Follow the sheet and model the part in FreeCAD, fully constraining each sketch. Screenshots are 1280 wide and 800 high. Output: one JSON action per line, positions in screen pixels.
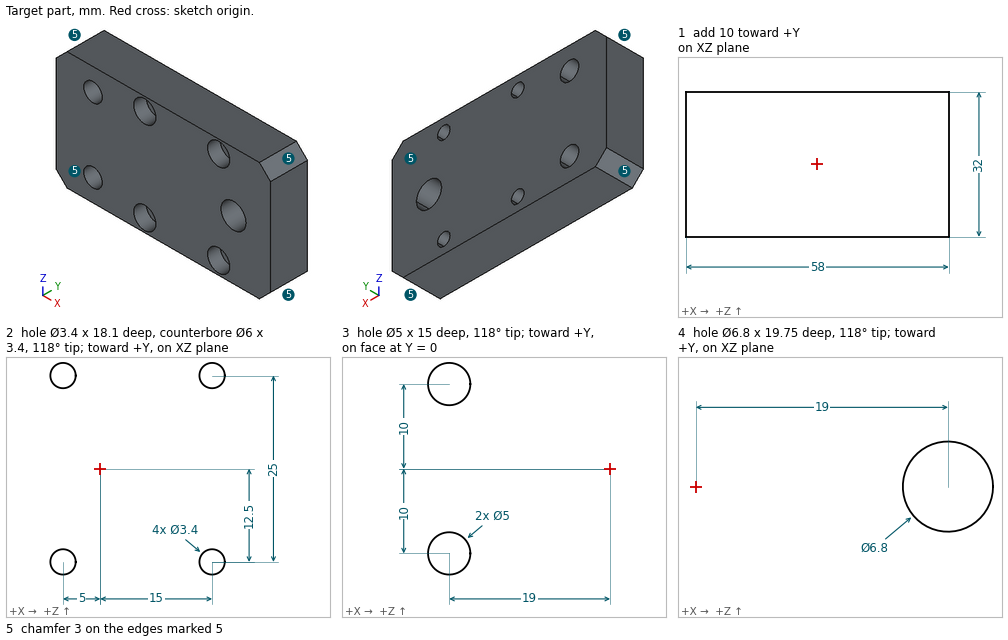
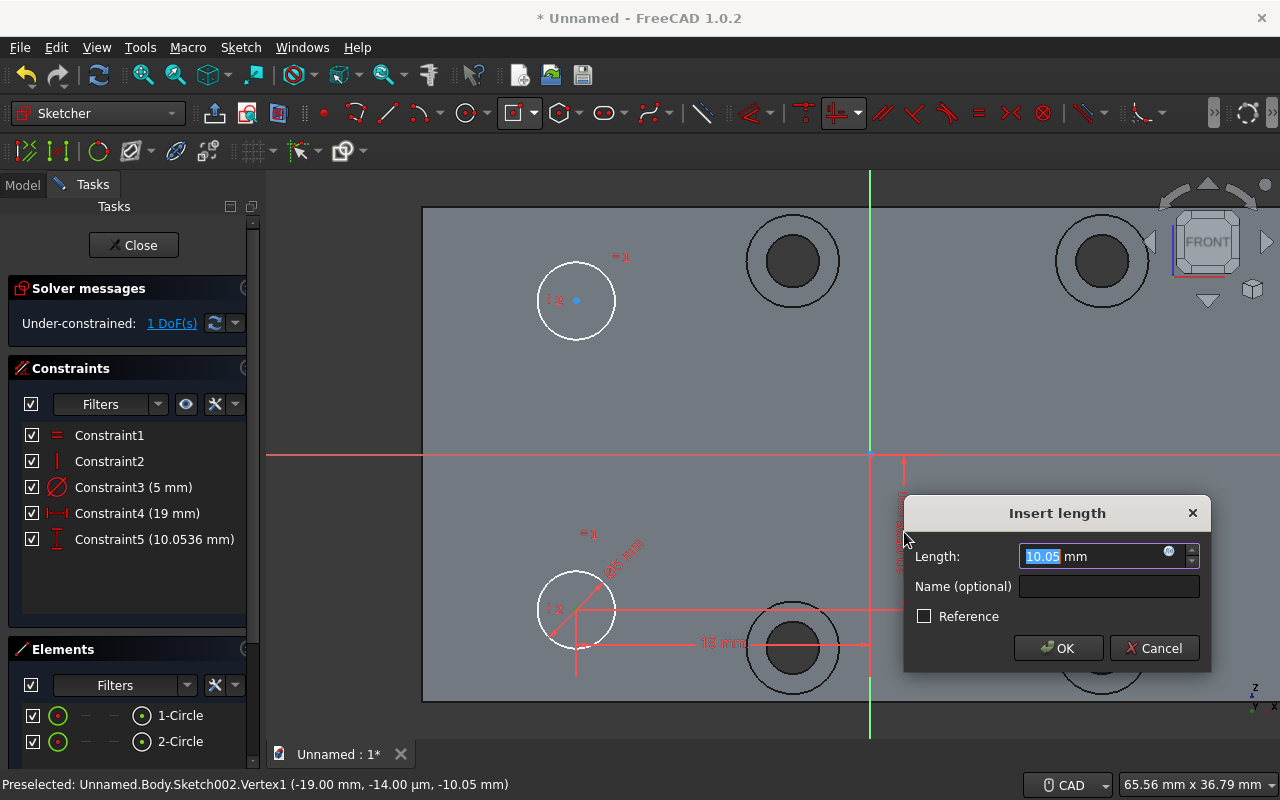
{"action": "type", "text": "10"}
{"action": "key", "text": "Return"}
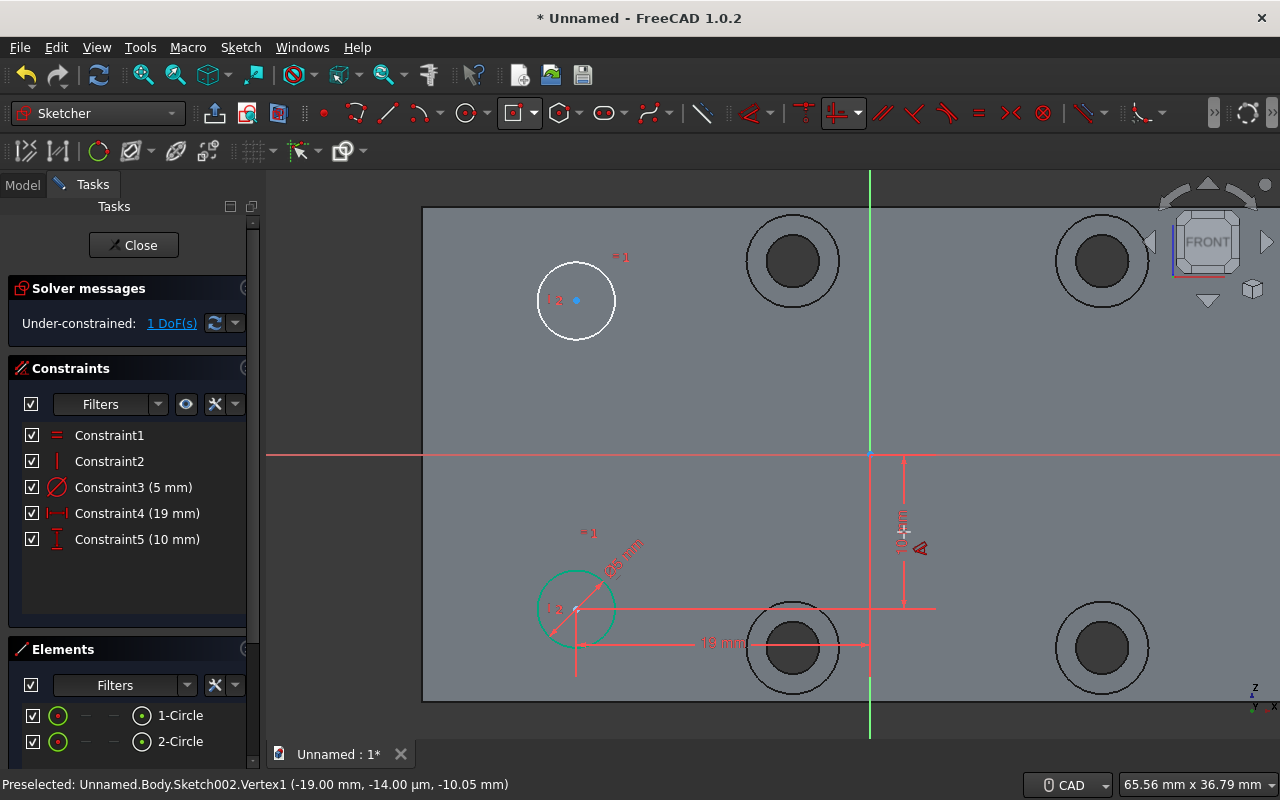
{"action": "left_click", "coordinate": [576, 301]}
{"action": "left_click", "coordinate": [904, 378]}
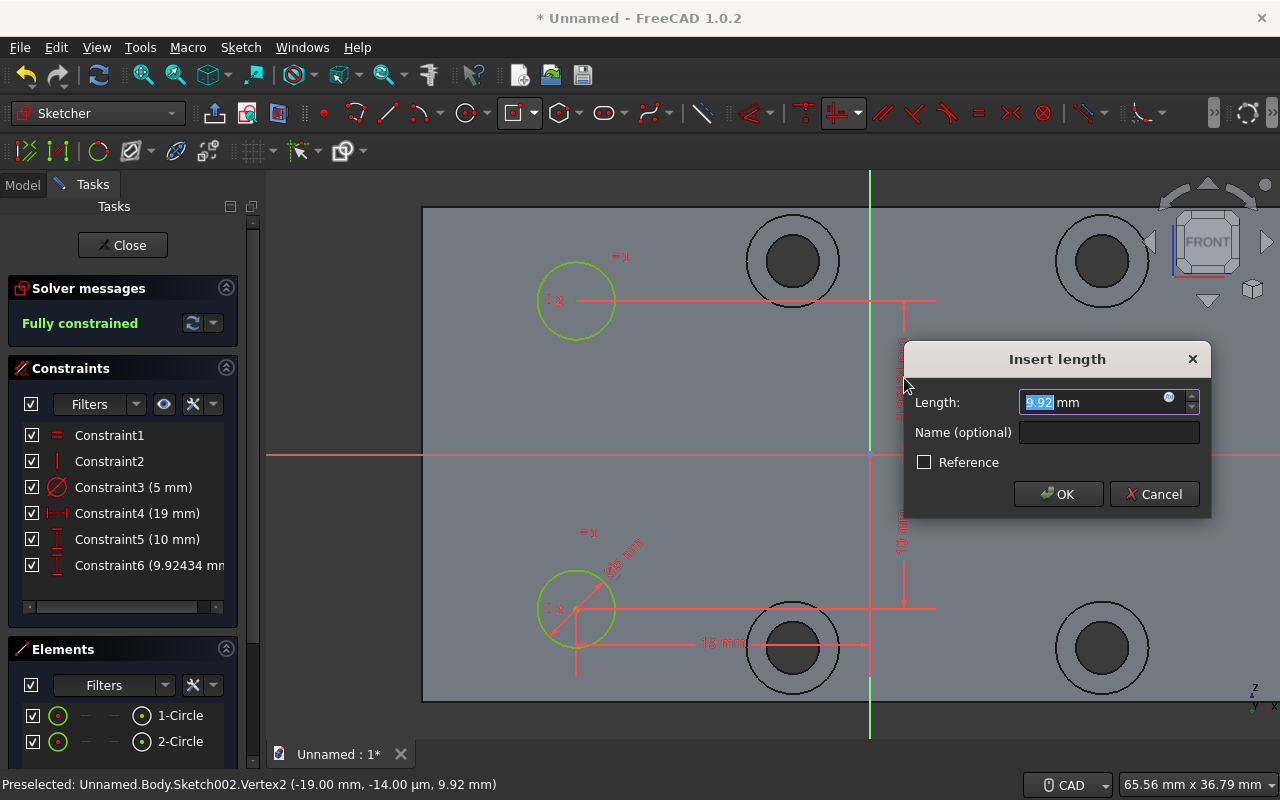
{"action": "type", "text": "10"}
{"action": "key", "text": "Return"}
{"action": "key", "text": "Escape"}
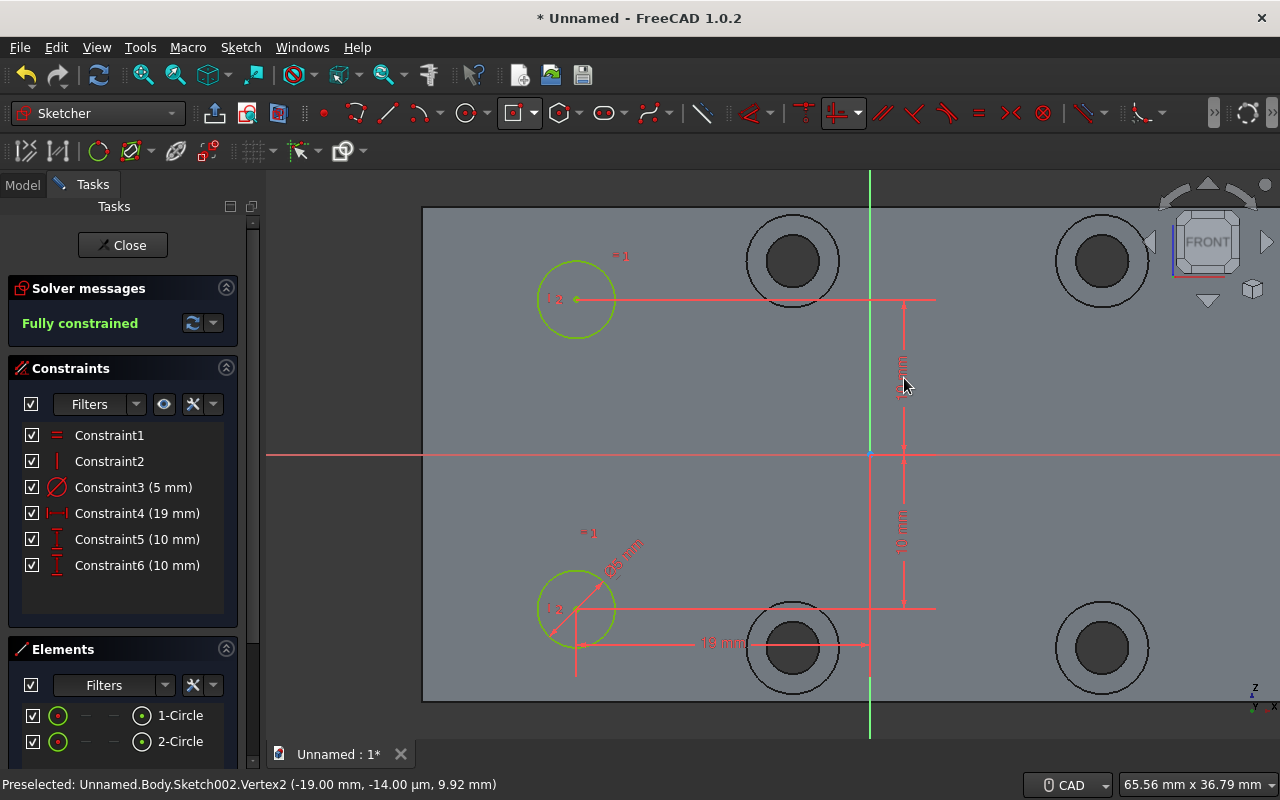
{"action": "left_click", "coordinate": [123, 245]}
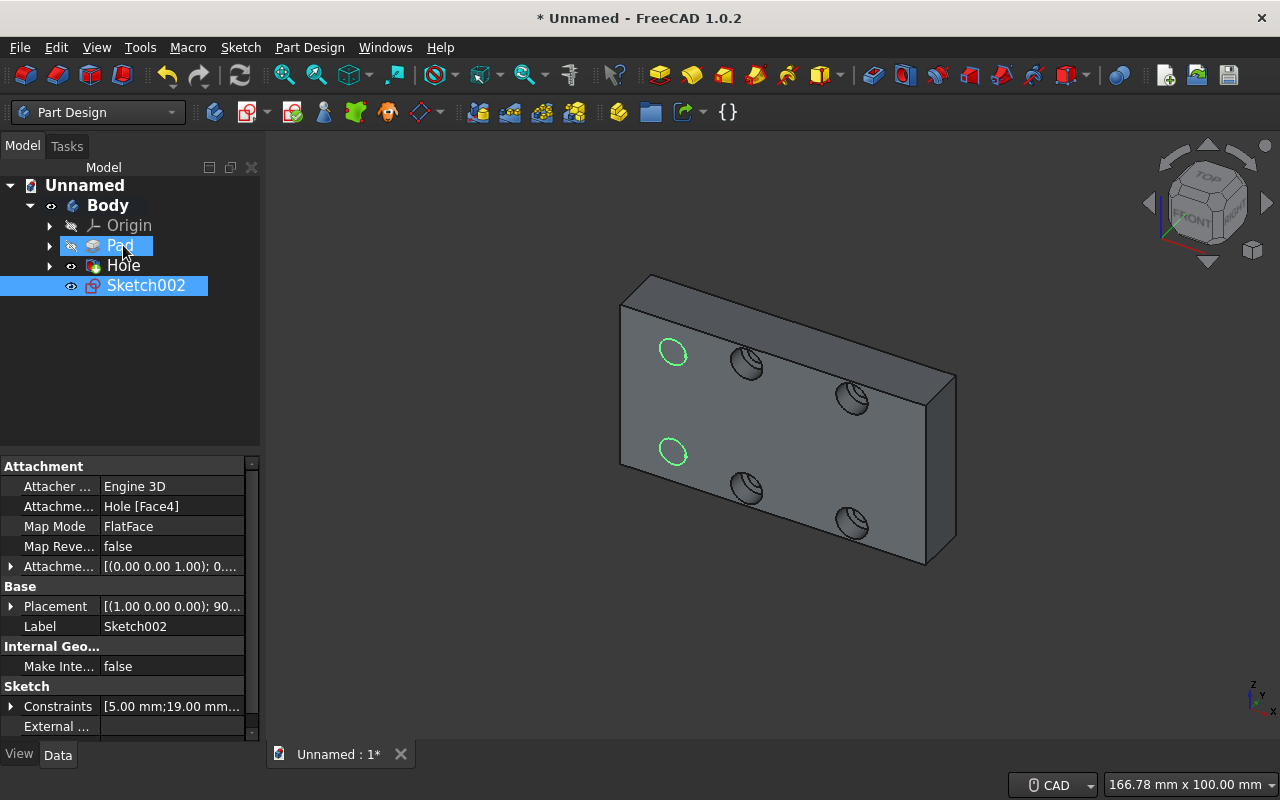
{"action": "left_click", "coordinate": [906, 76]}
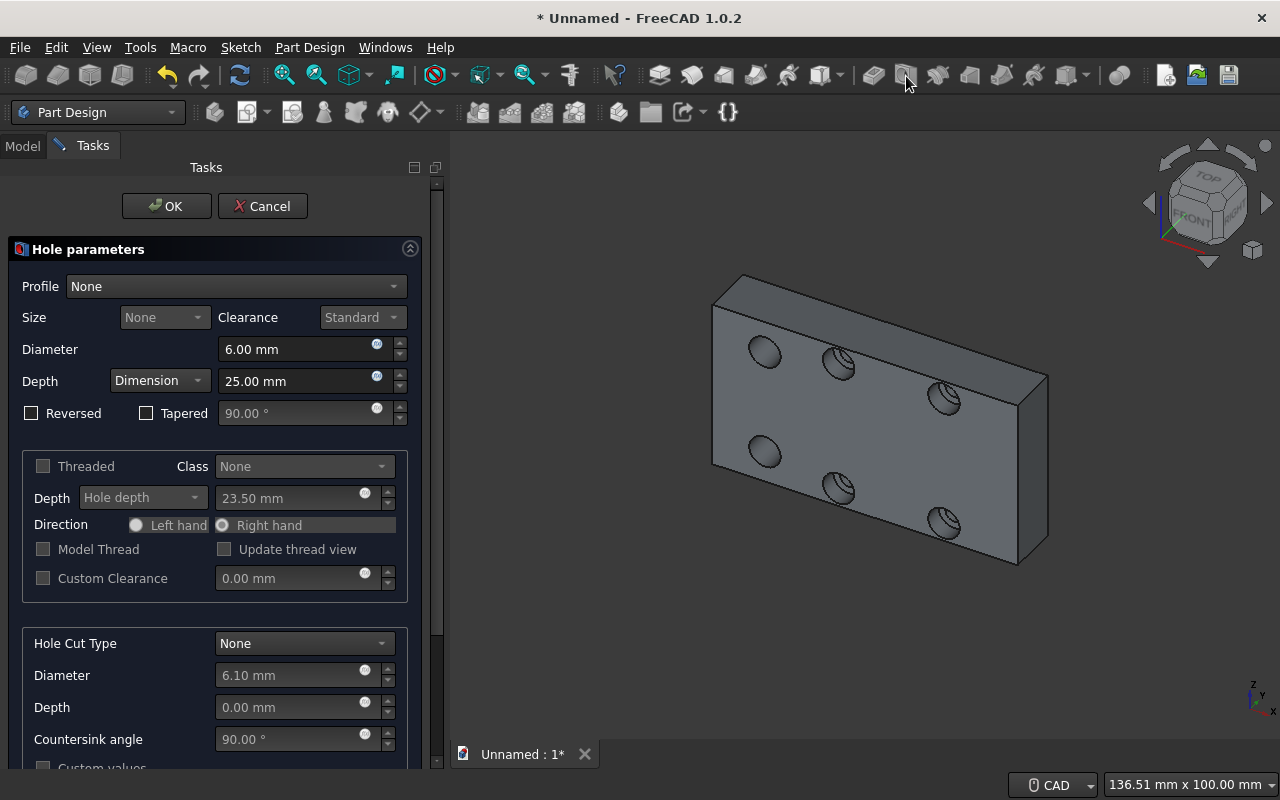
{"action": "triple_click", "coordinate": [305, 349]}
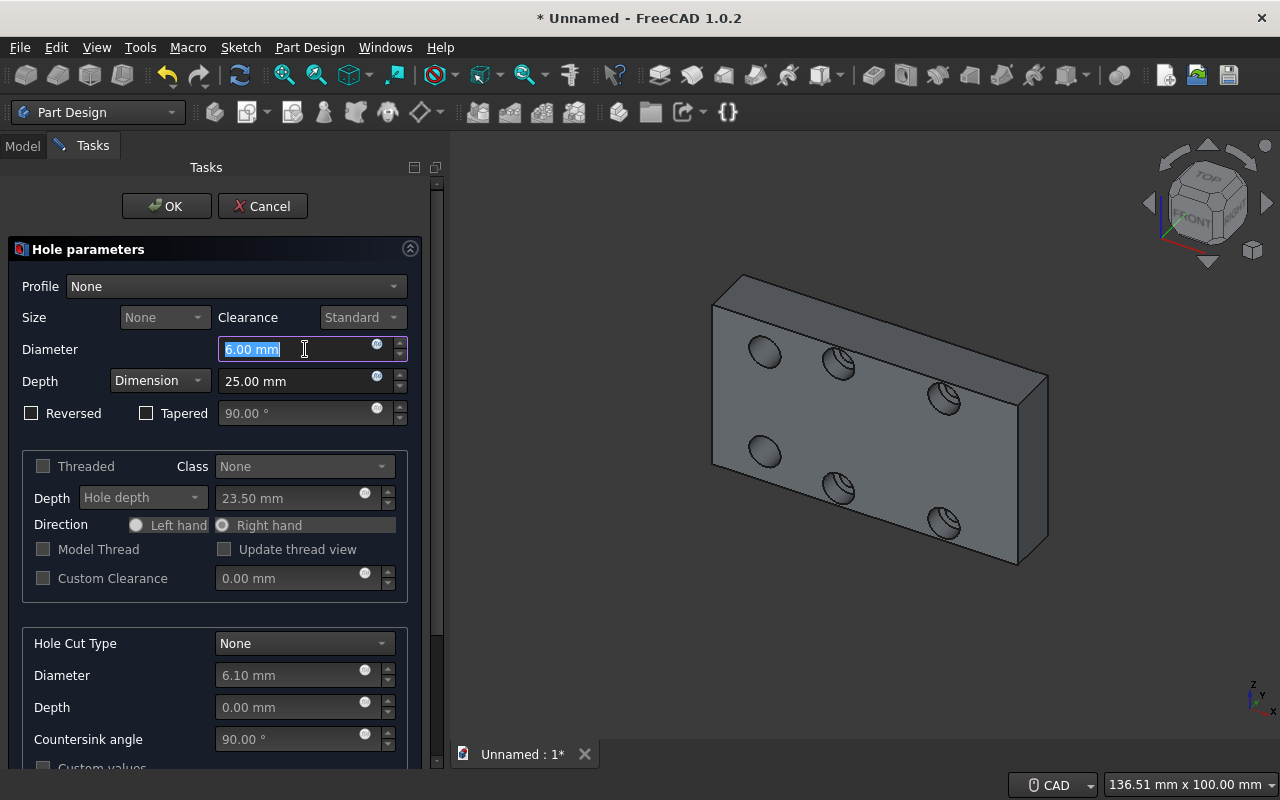
{"action": "type", "text": "5"}
{"action": "key", "text": "Tab"}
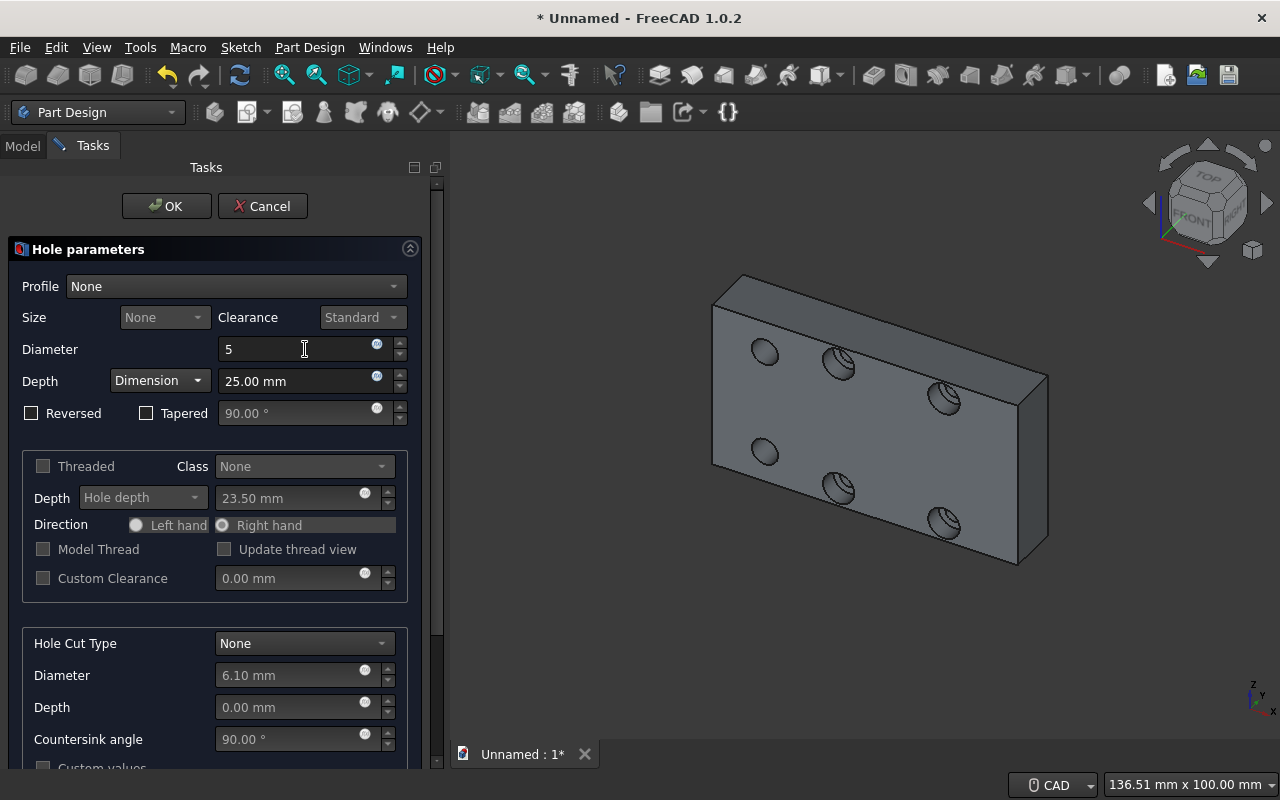
{"action": "triple_click", "coordinate": [305, 381]}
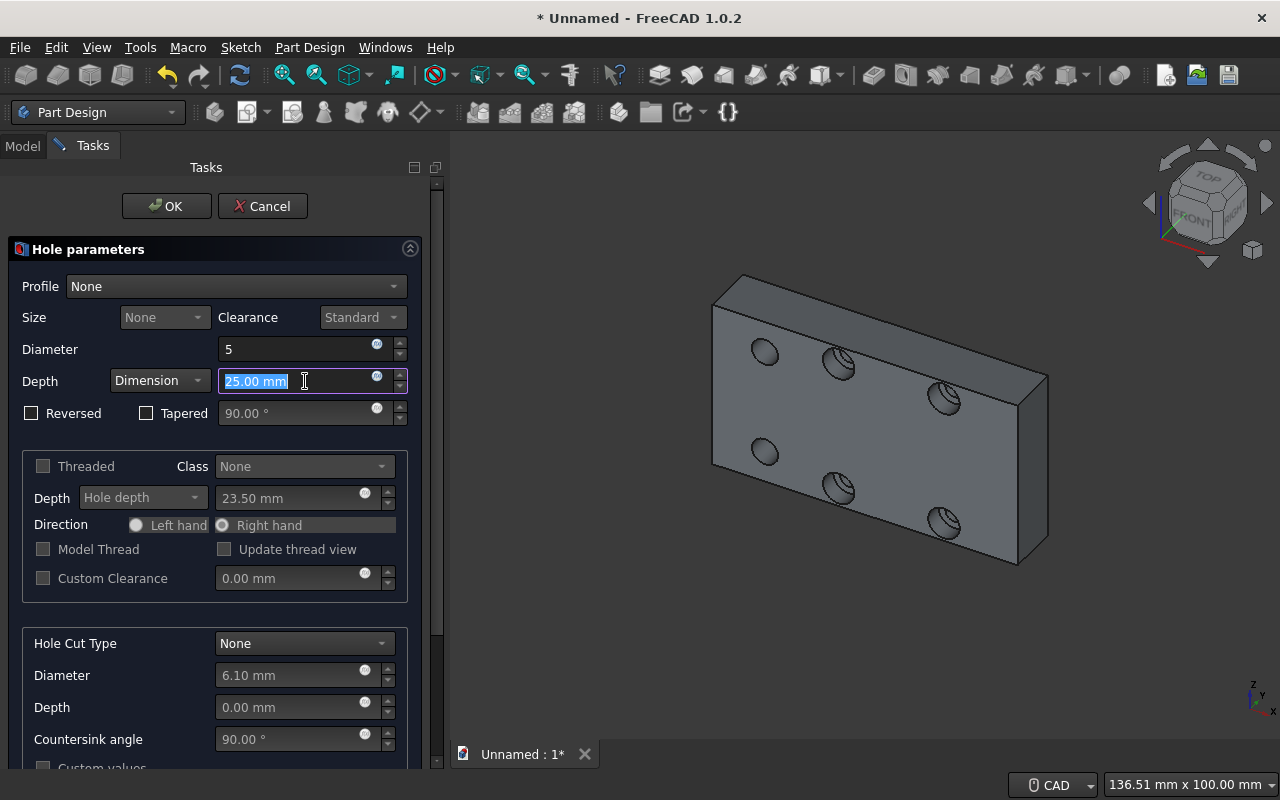
{"action": "type", "text": "15"}
{"action": "key", "text": "Tab"}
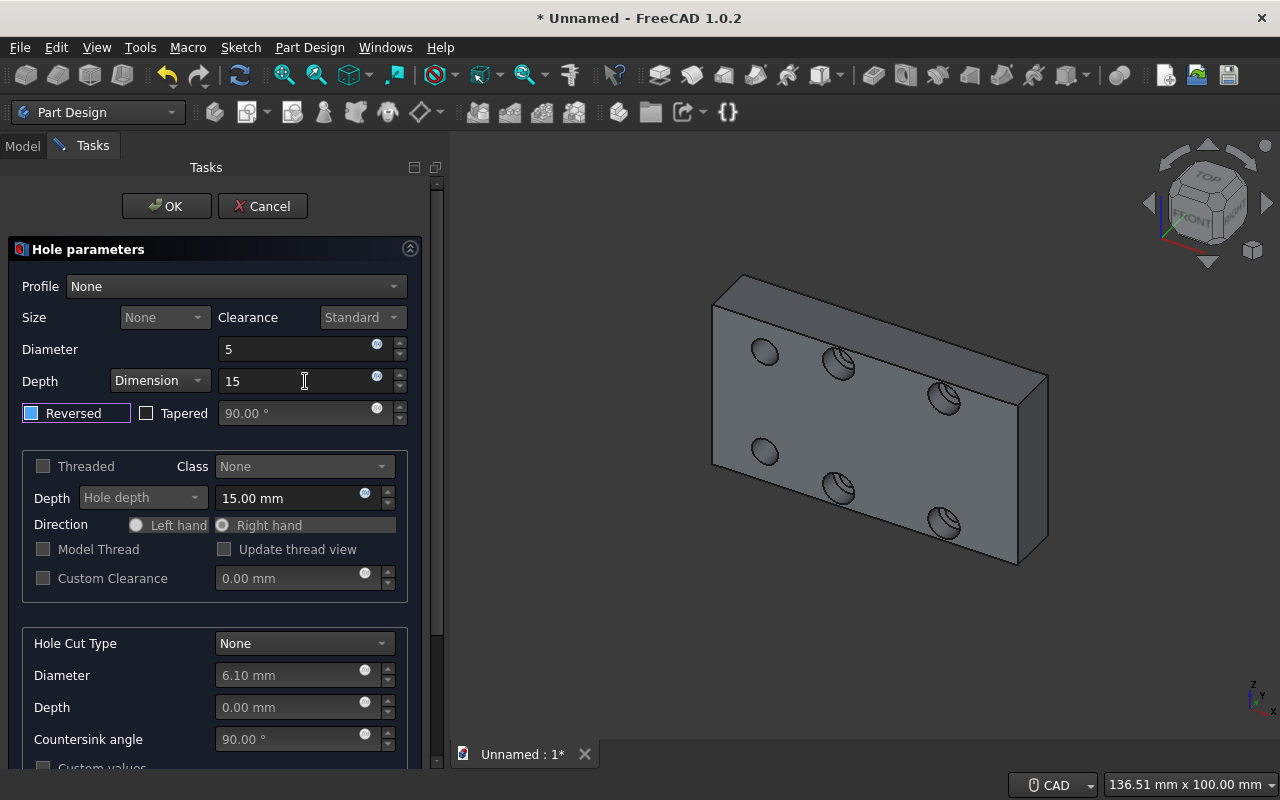
{"action": "left_click", "coordinate": [167, 206]}